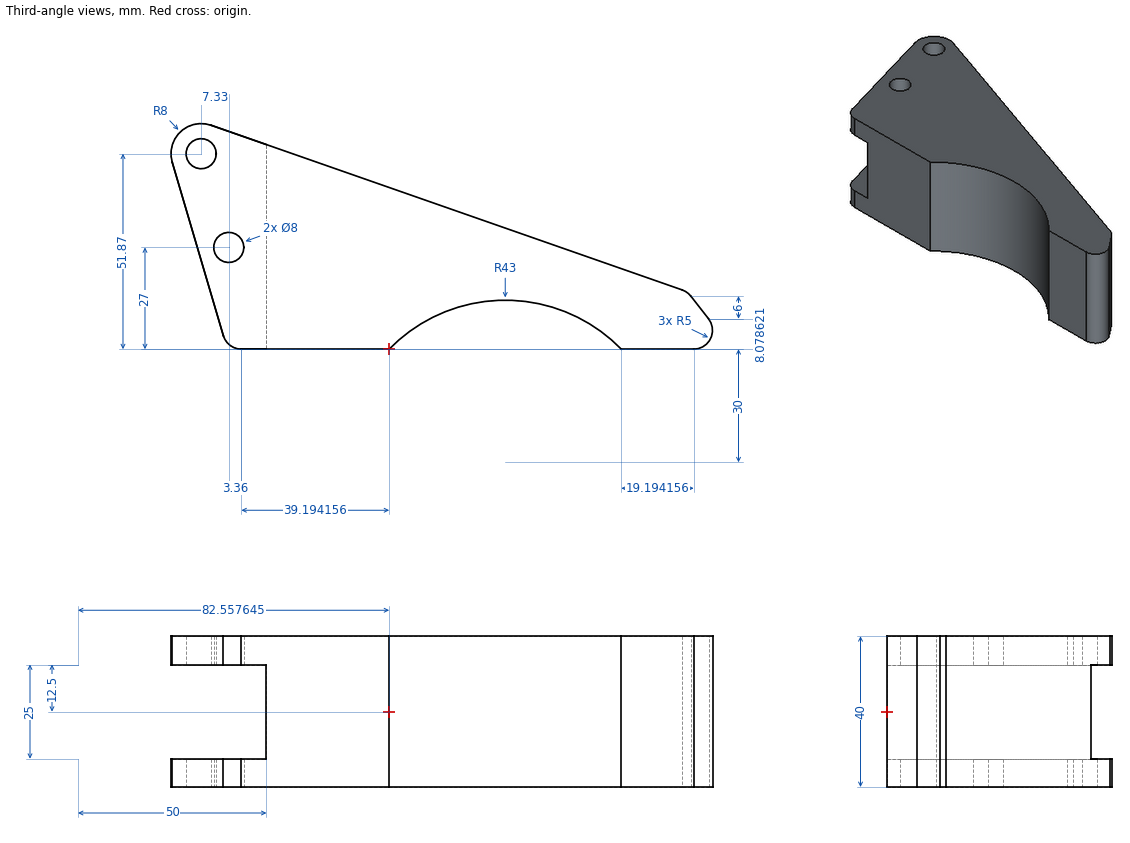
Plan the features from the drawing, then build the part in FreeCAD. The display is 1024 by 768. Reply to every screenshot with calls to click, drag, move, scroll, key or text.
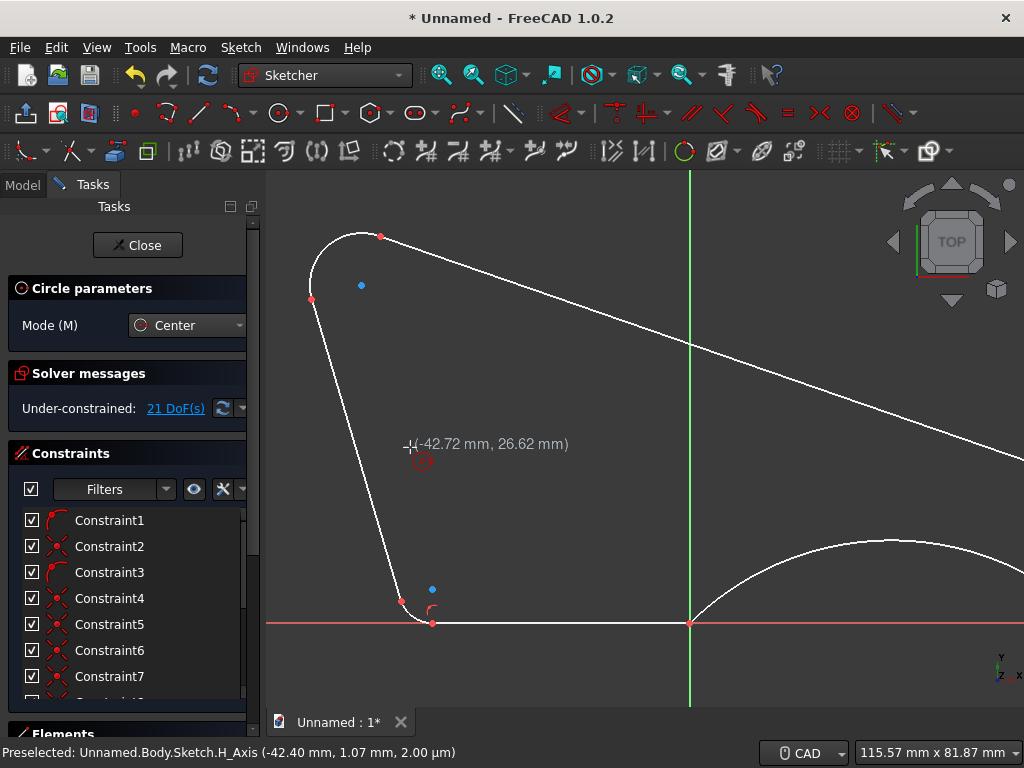
click(411, 446)
click(429, 428)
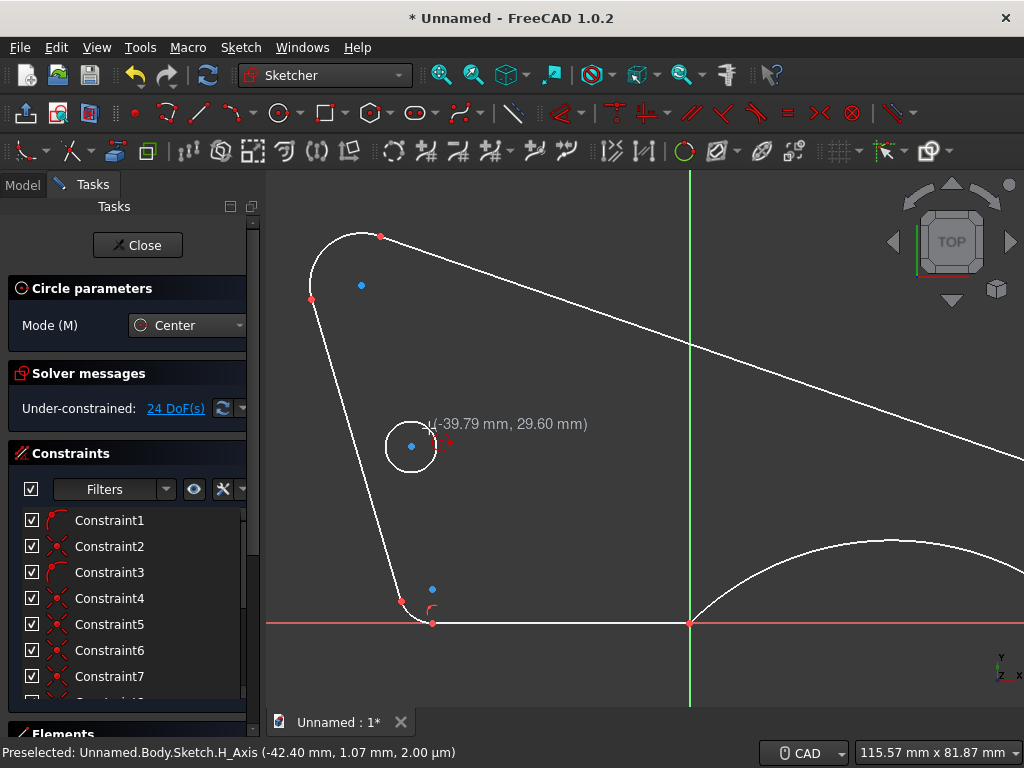
click(363, 283)
click(381, 264)
key(Escape)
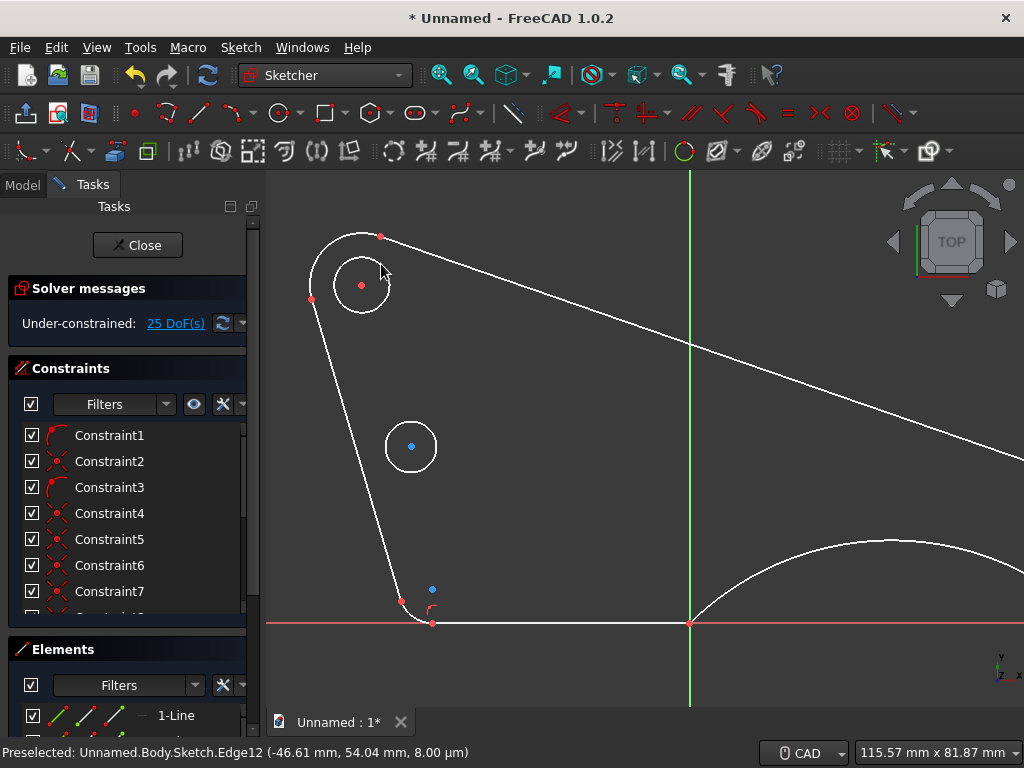
click(509, 623)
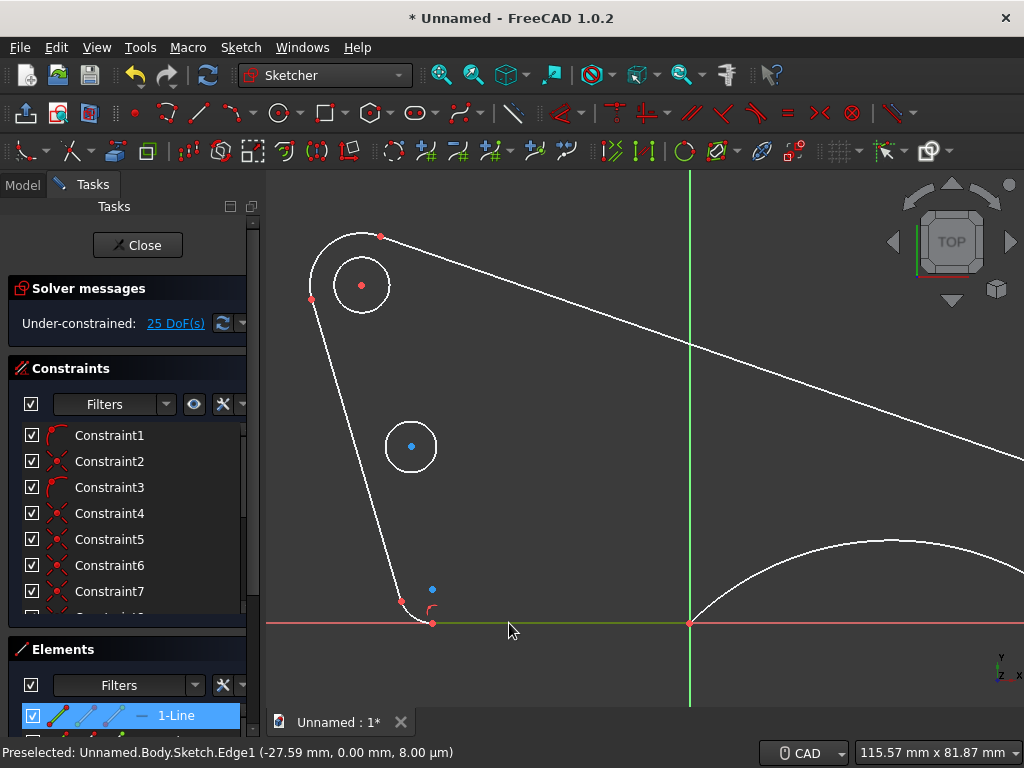
click(407, 612)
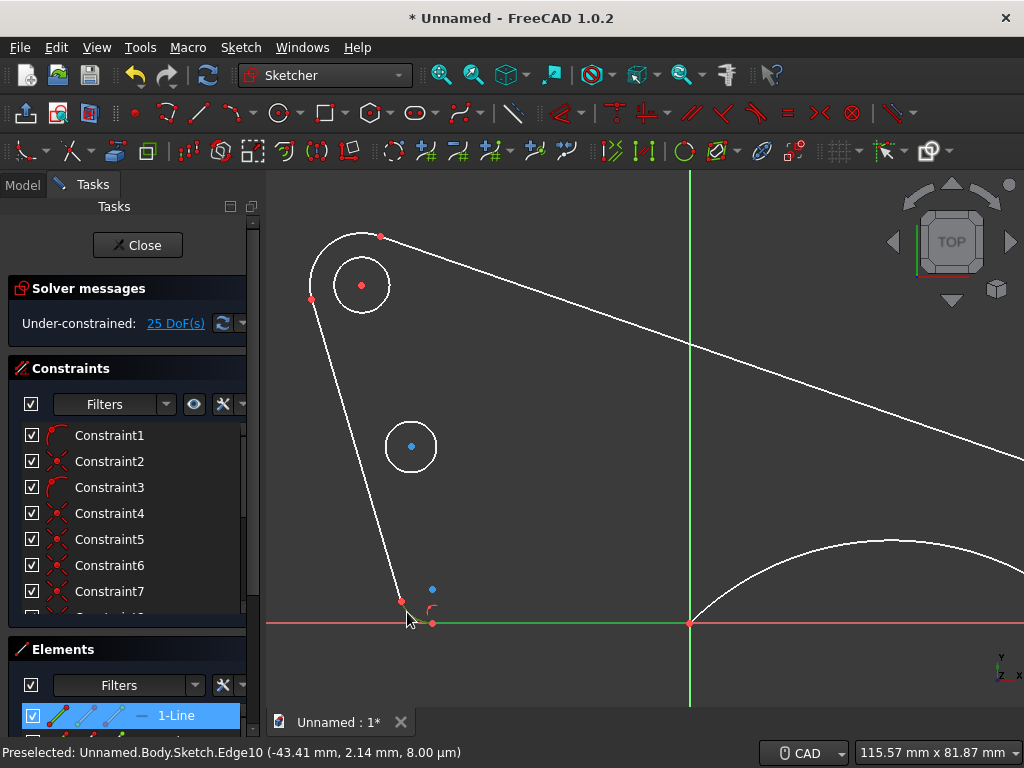
click(756, 114)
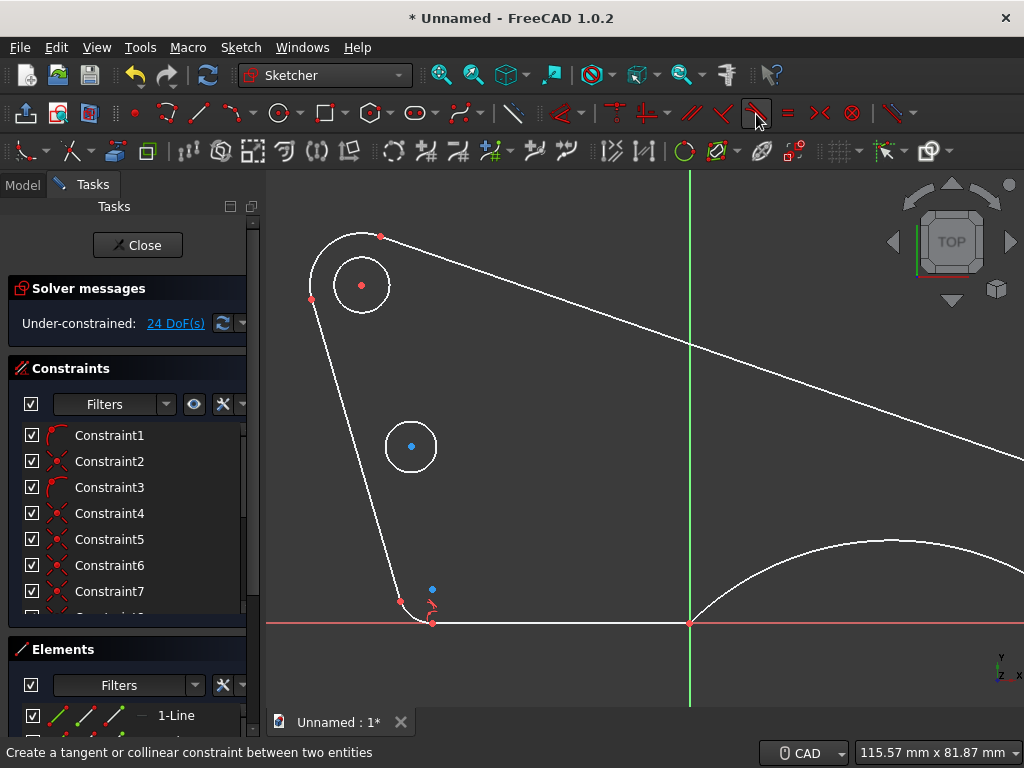
scroll(410, 447, down, 4)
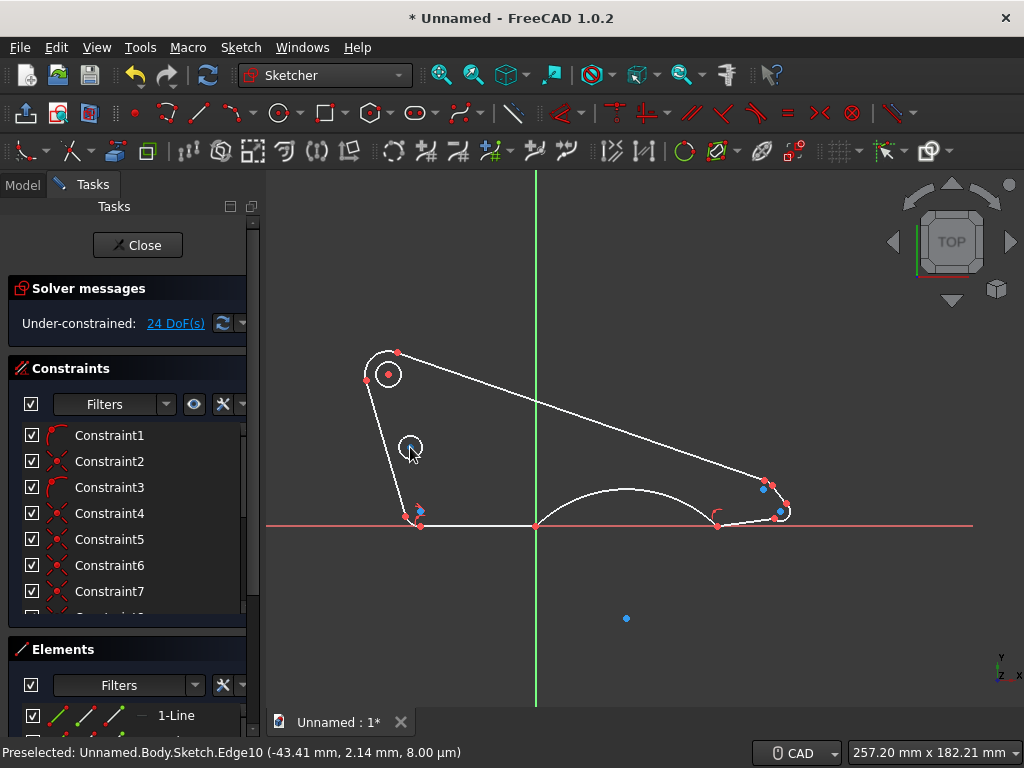
scroll(757, 521, up, 5)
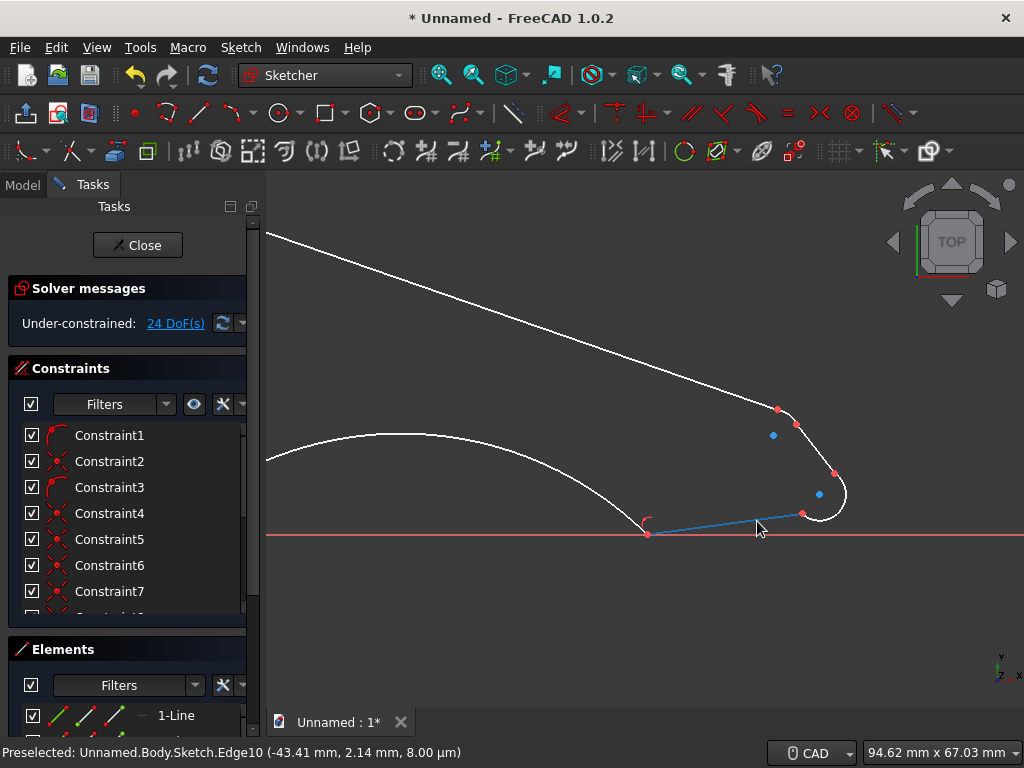
click(756, 520)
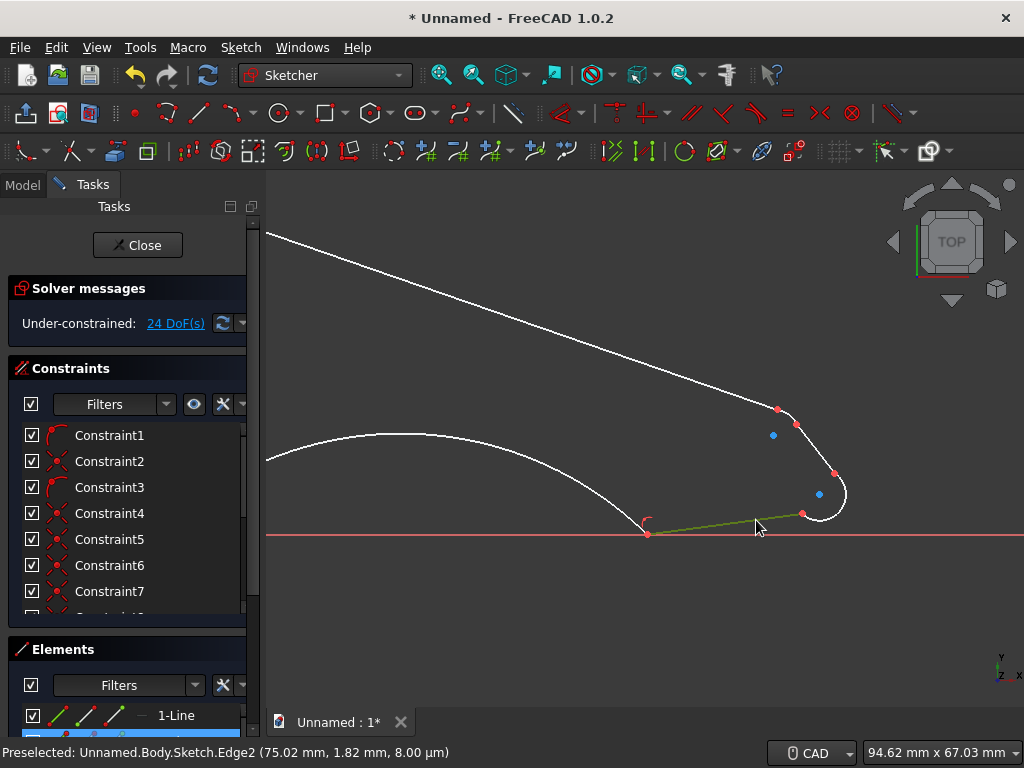
click(826, 520)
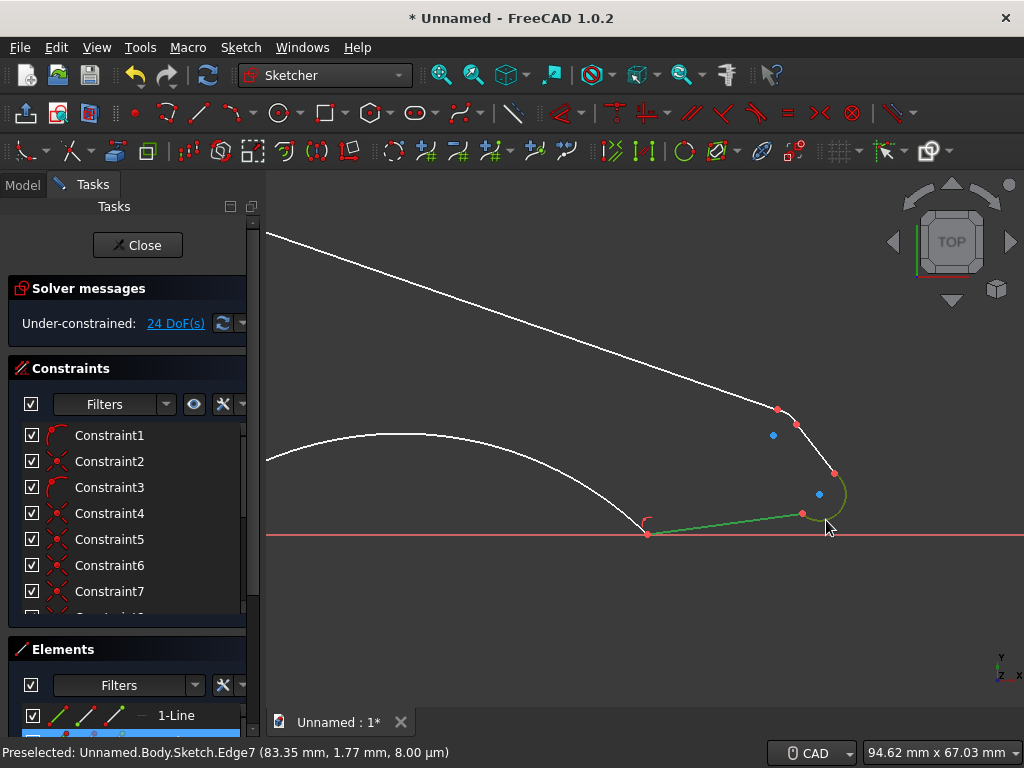
click(756, 114)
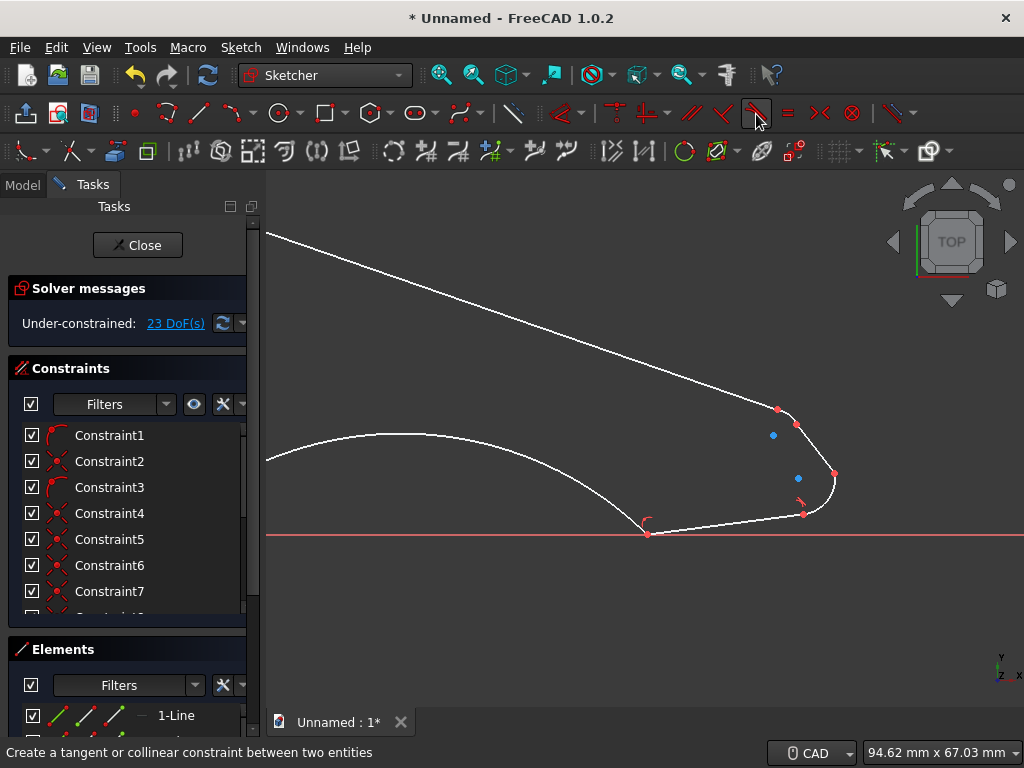
click(823, 458)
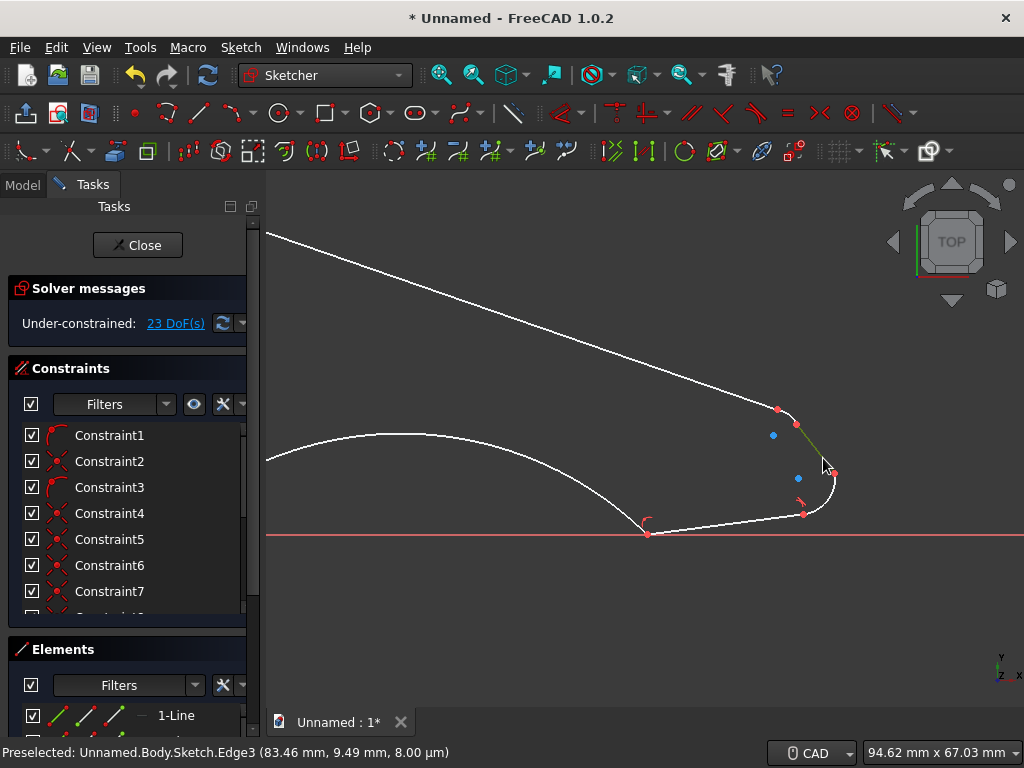
click(819, 508)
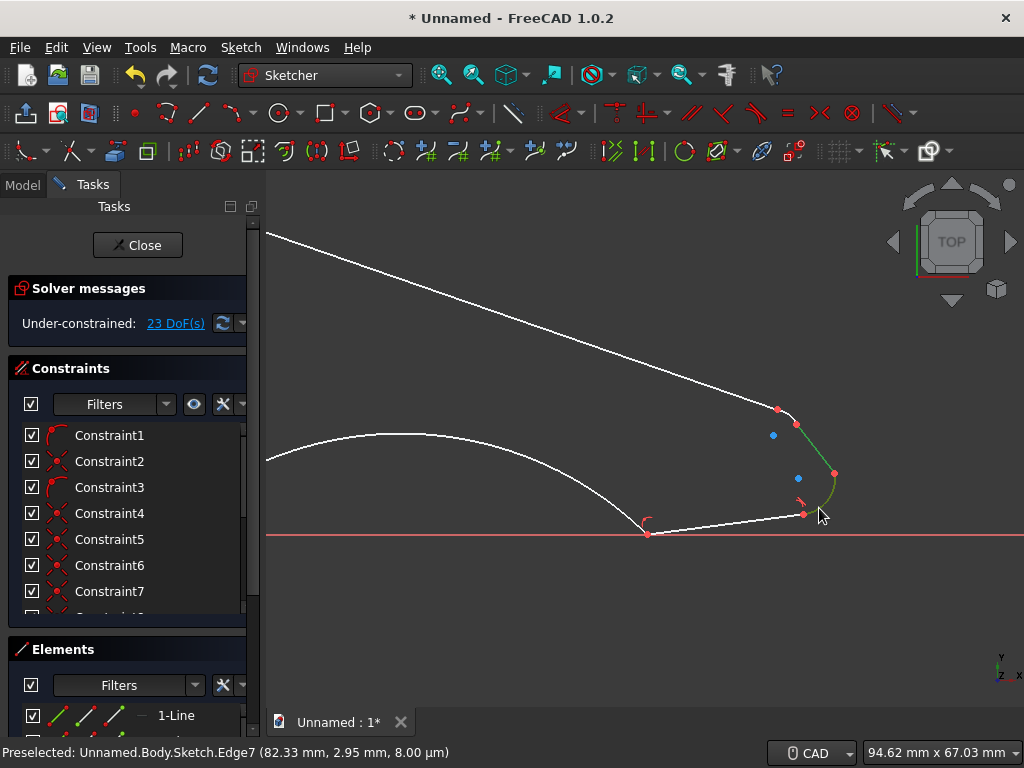
click(756, 114)